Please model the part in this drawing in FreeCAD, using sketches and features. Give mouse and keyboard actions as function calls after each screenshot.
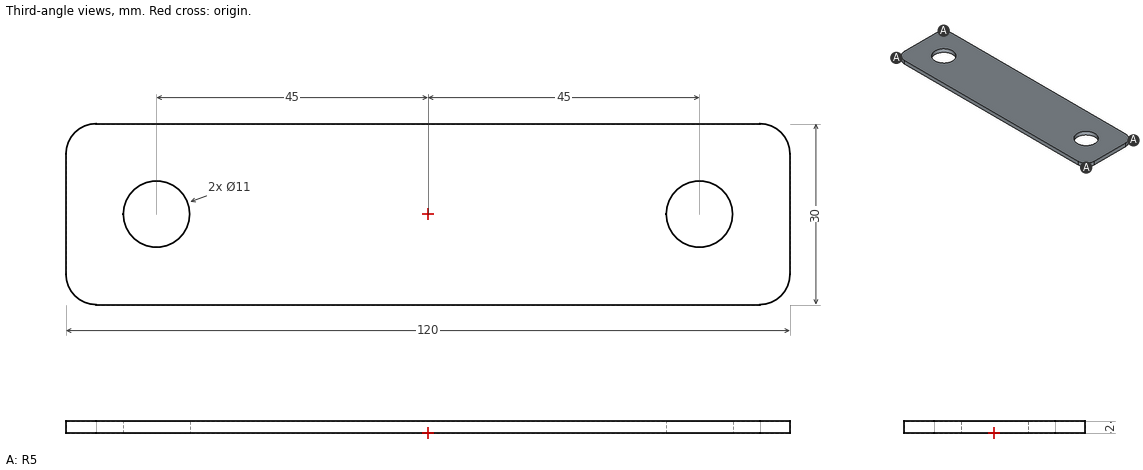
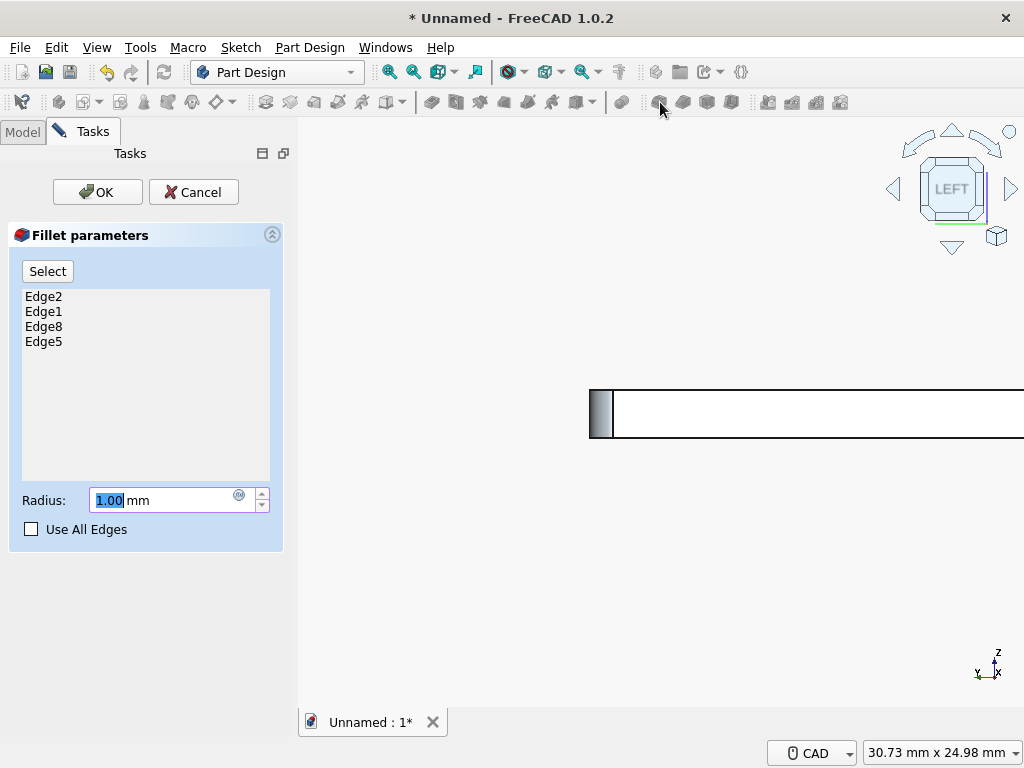
text(5)
key(Tab)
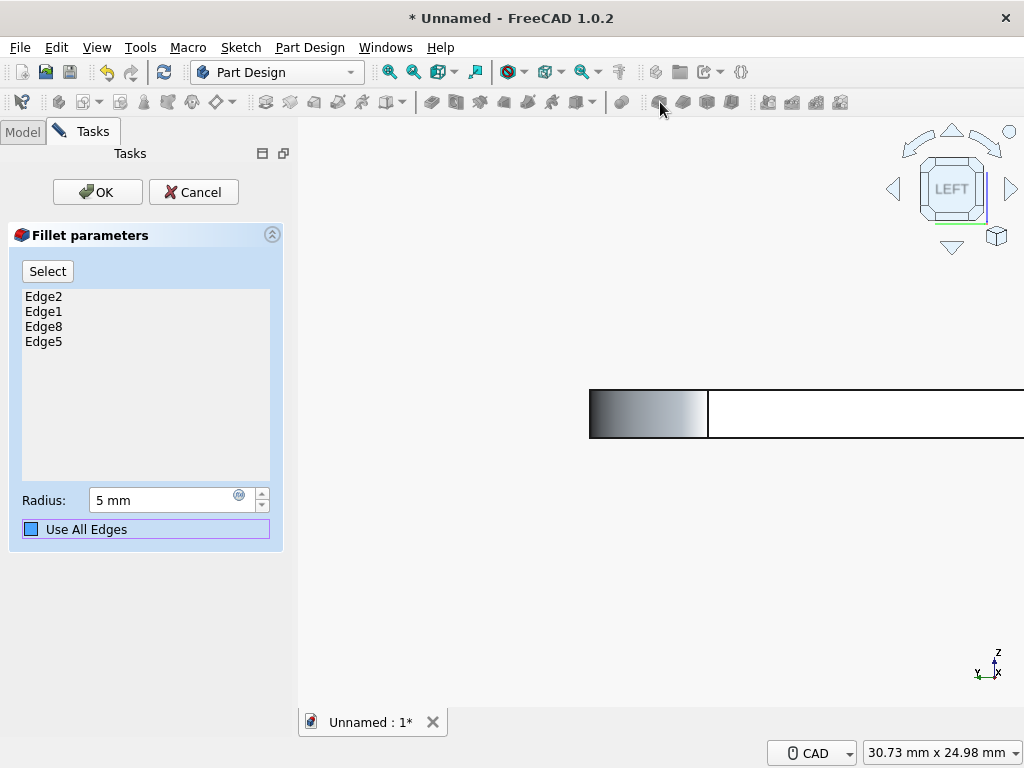
click(98, 192)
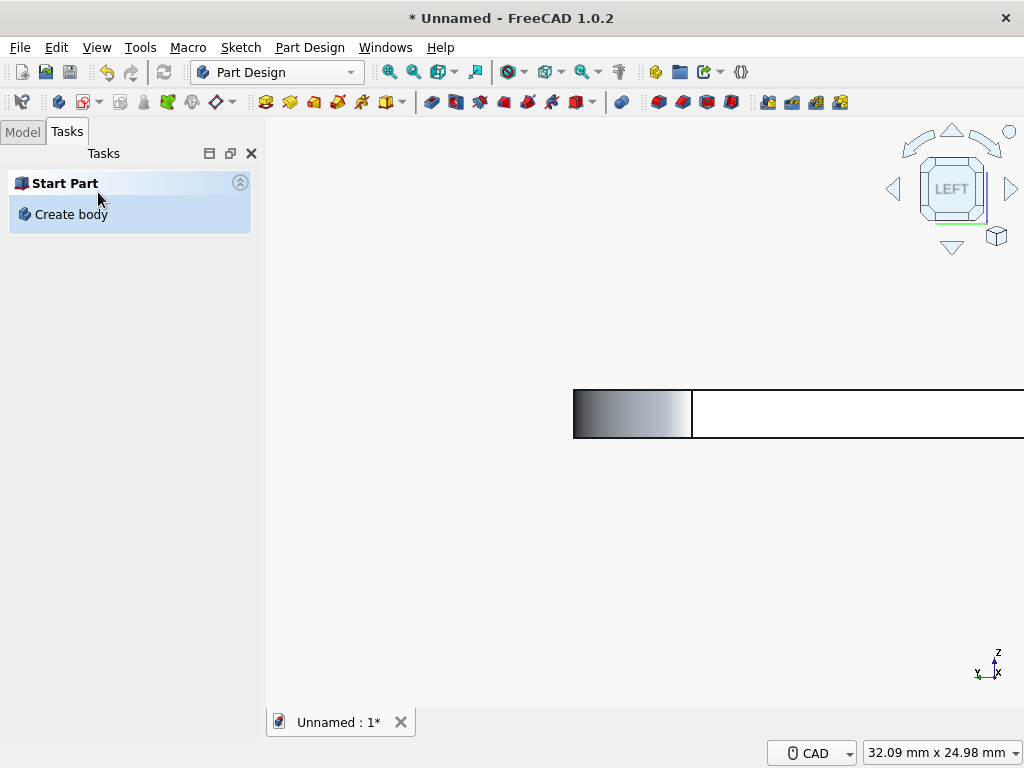
key(0)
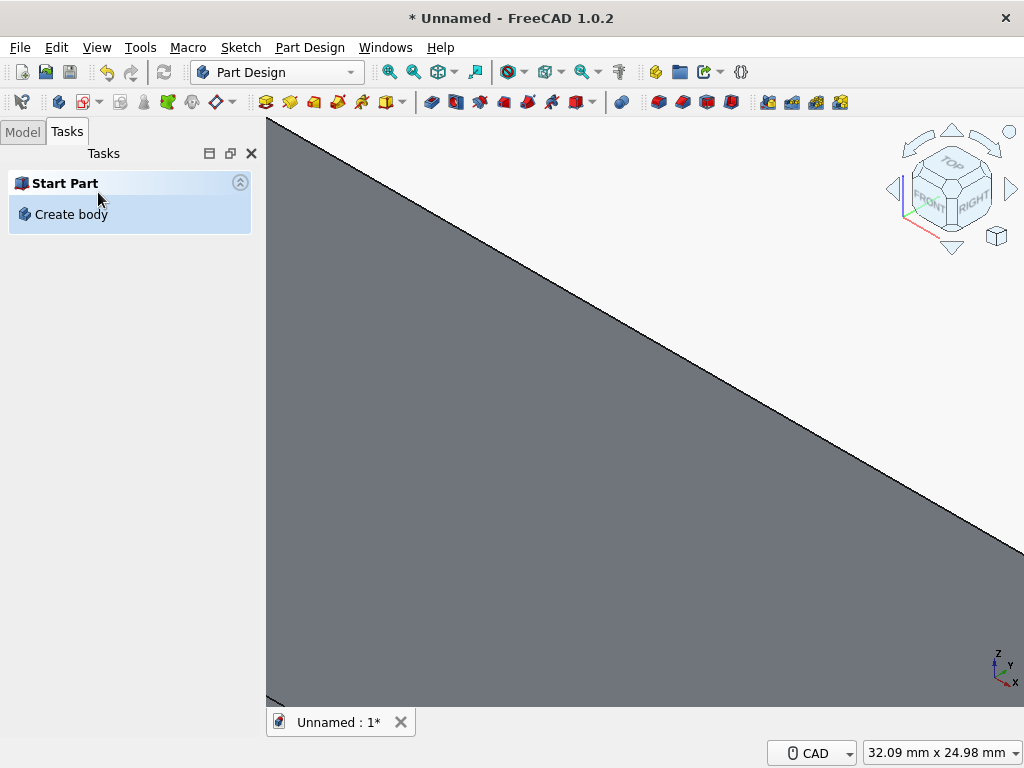
click(390, 72)